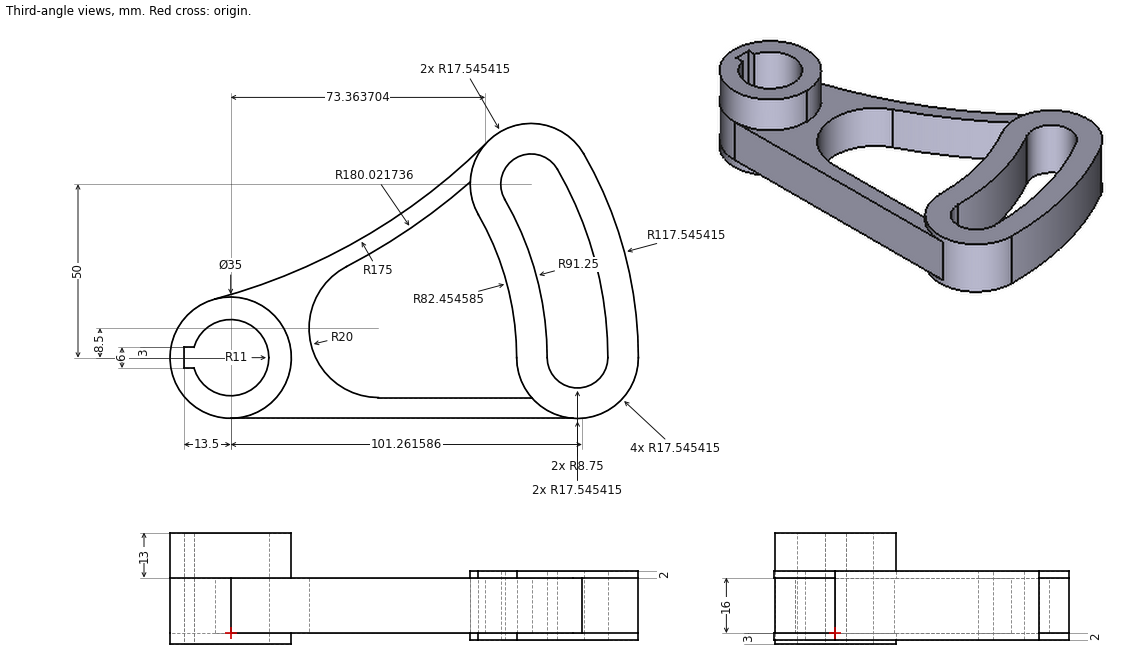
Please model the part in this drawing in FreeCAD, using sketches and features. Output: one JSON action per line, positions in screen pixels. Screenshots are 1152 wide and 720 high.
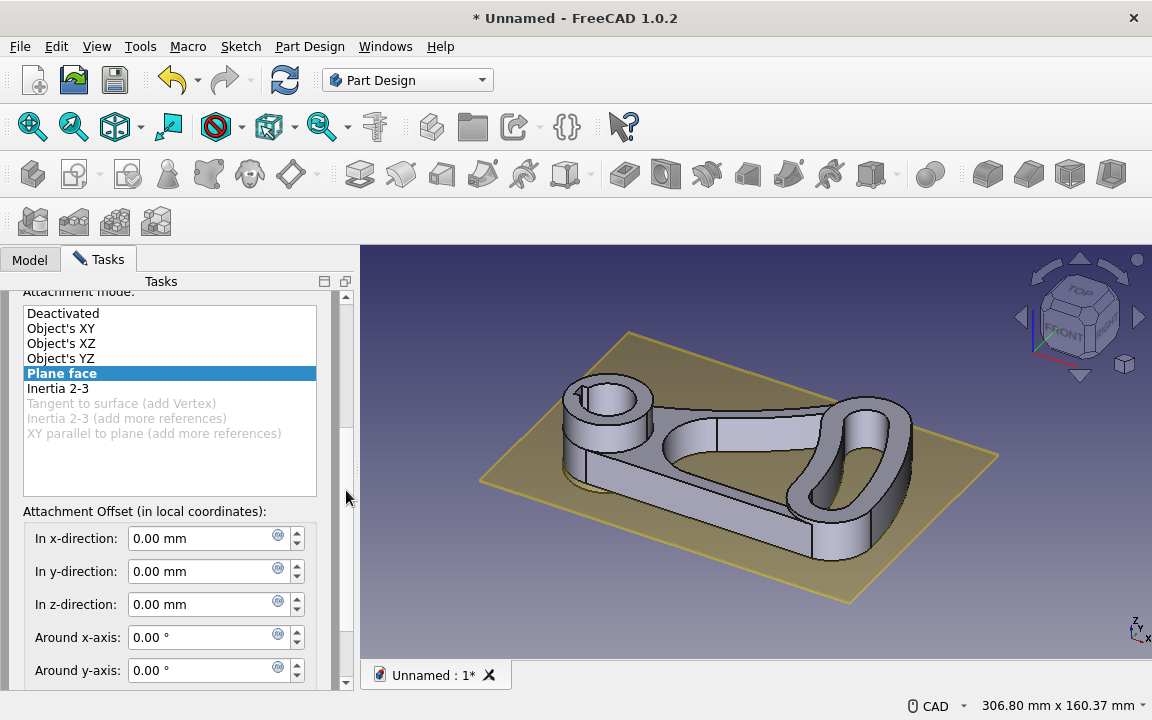
{"action": "triple_click", "coordinate": [210, 604]}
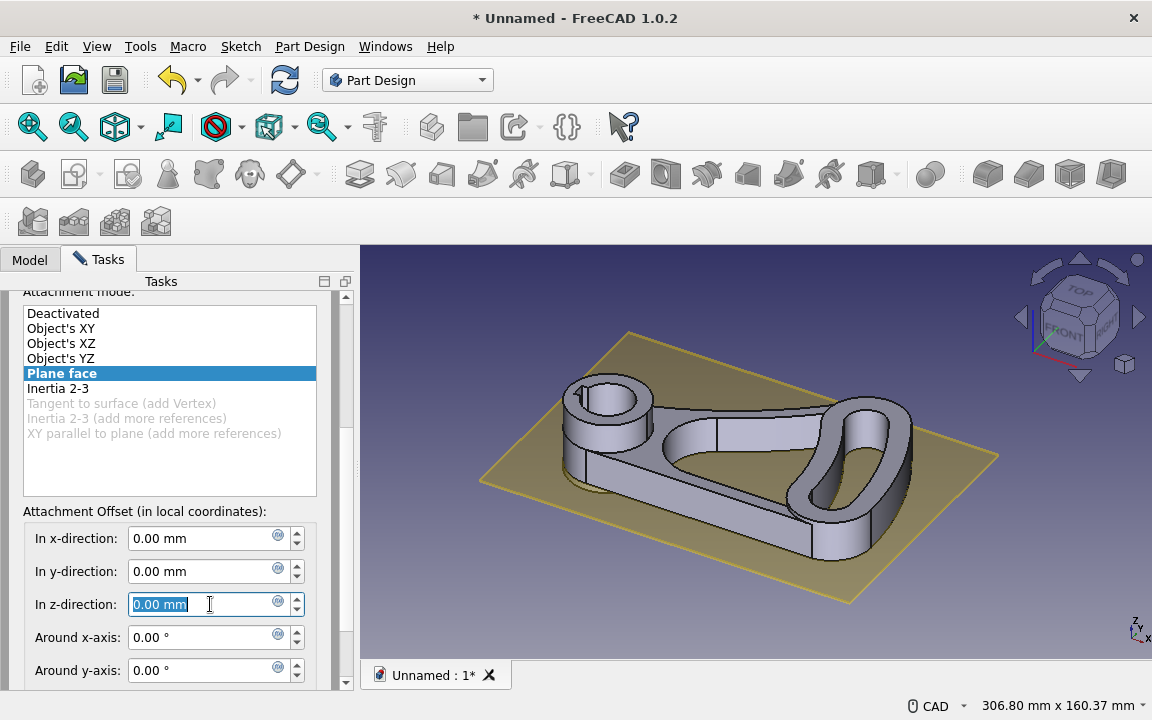
{"action": "type", "text": "-2"}
{"action": "key", "text": "Tab"}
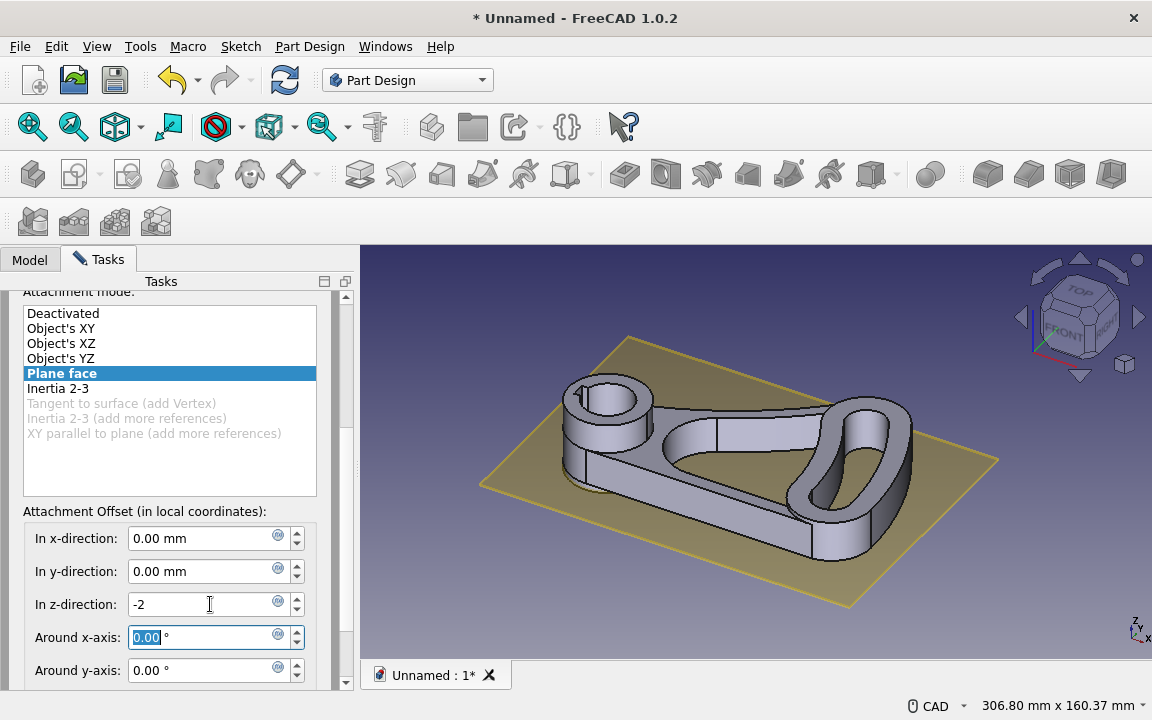
{"action": "scroll", "coordinate": [346, 490], "scroll_direction": "up", "scroll_amount": 5}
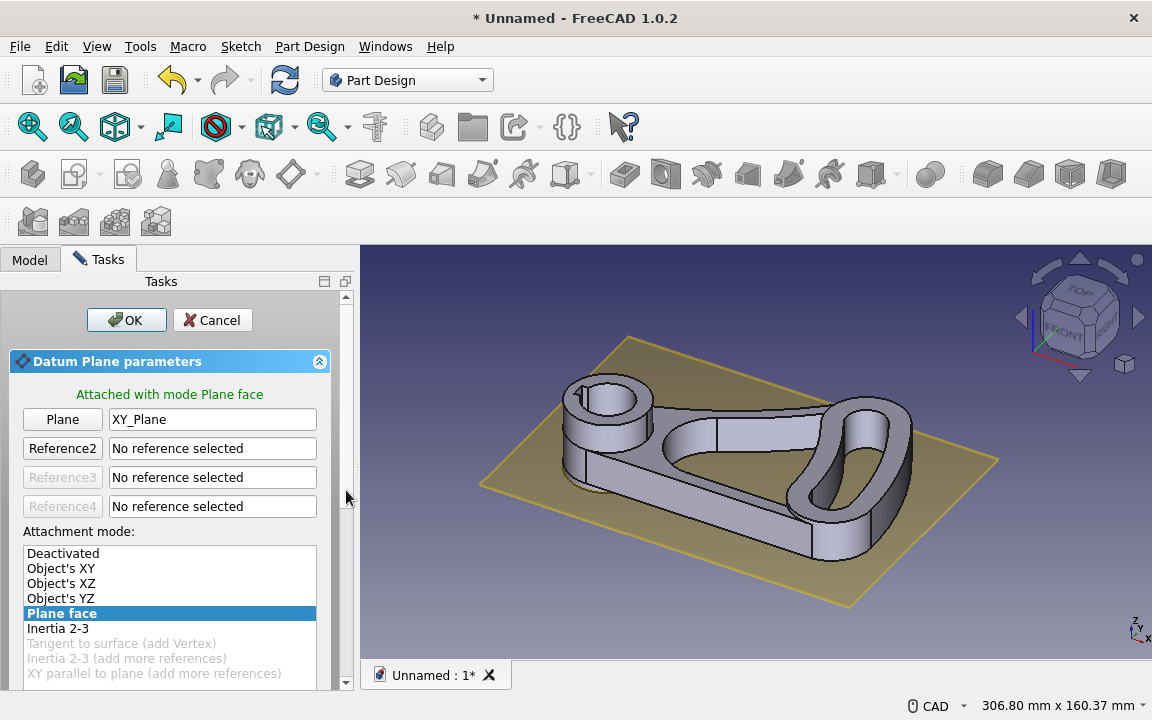
{"action": "left_click", "coordinate": [127, 320]}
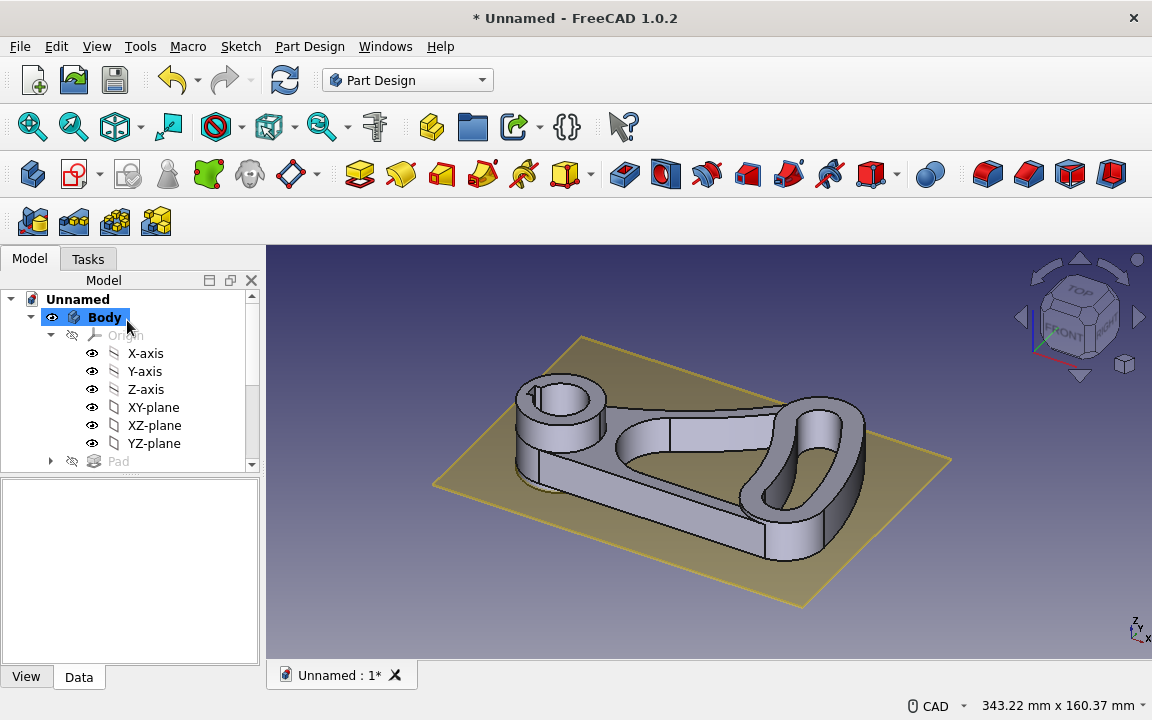
{"action": "scroll", "coordinate": [101, 385], "scroll_direction": "down", "scroll_amount": 3}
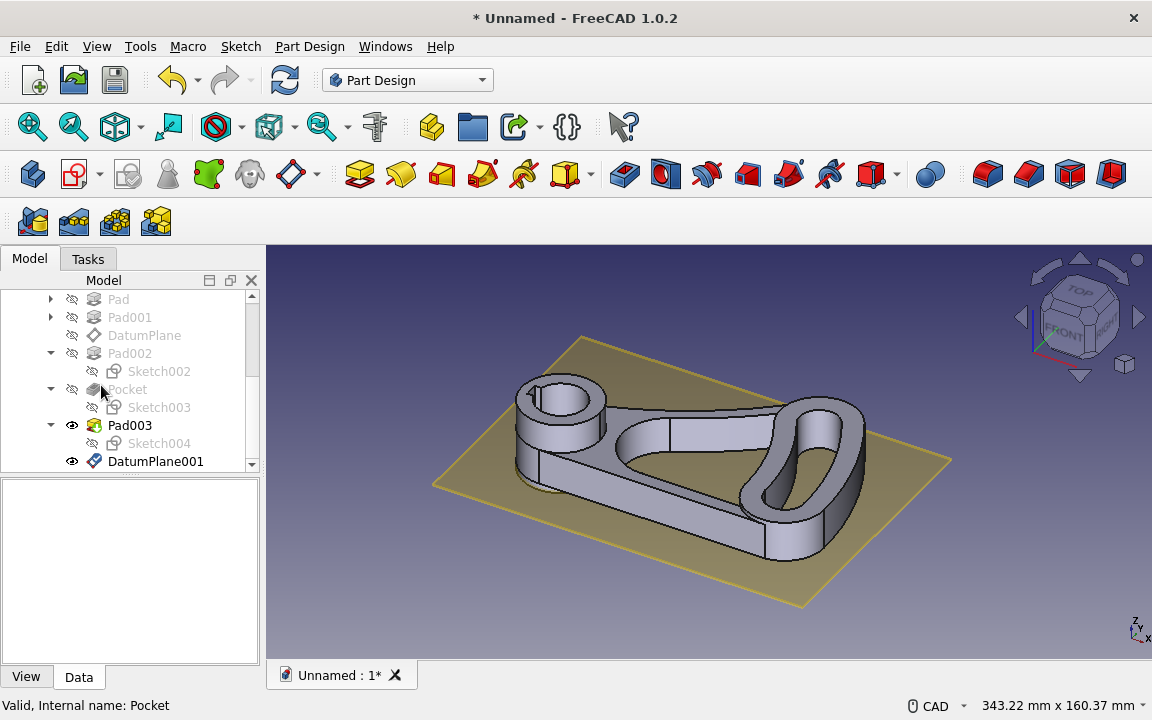
{"action": "left_click", "coordinate": [117, 461]}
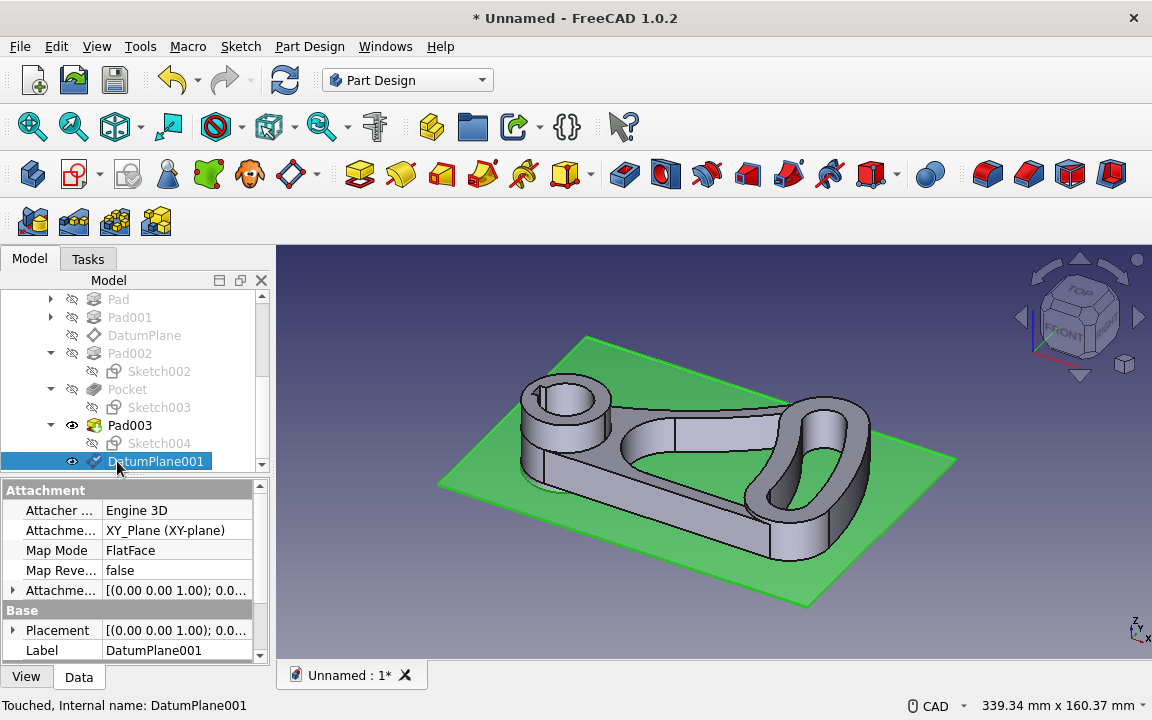
{"action": "left_click", "coordinate": [74, 174]}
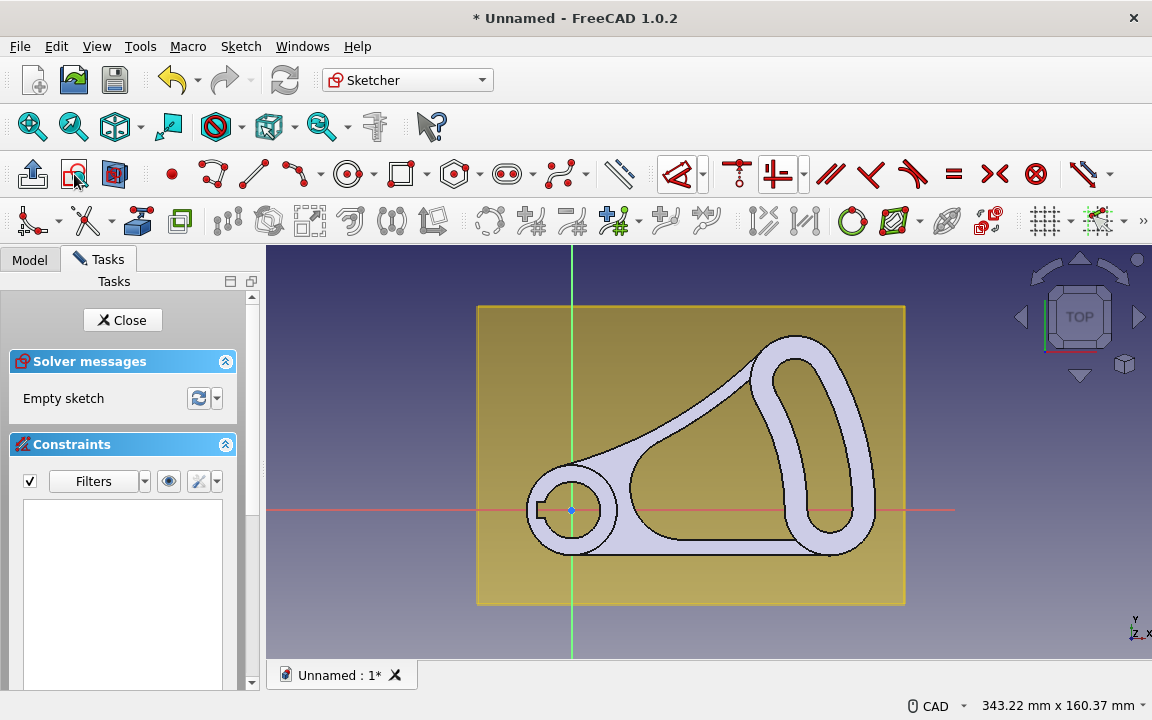
{"action": "left_click", "coordinate": [115, 174]}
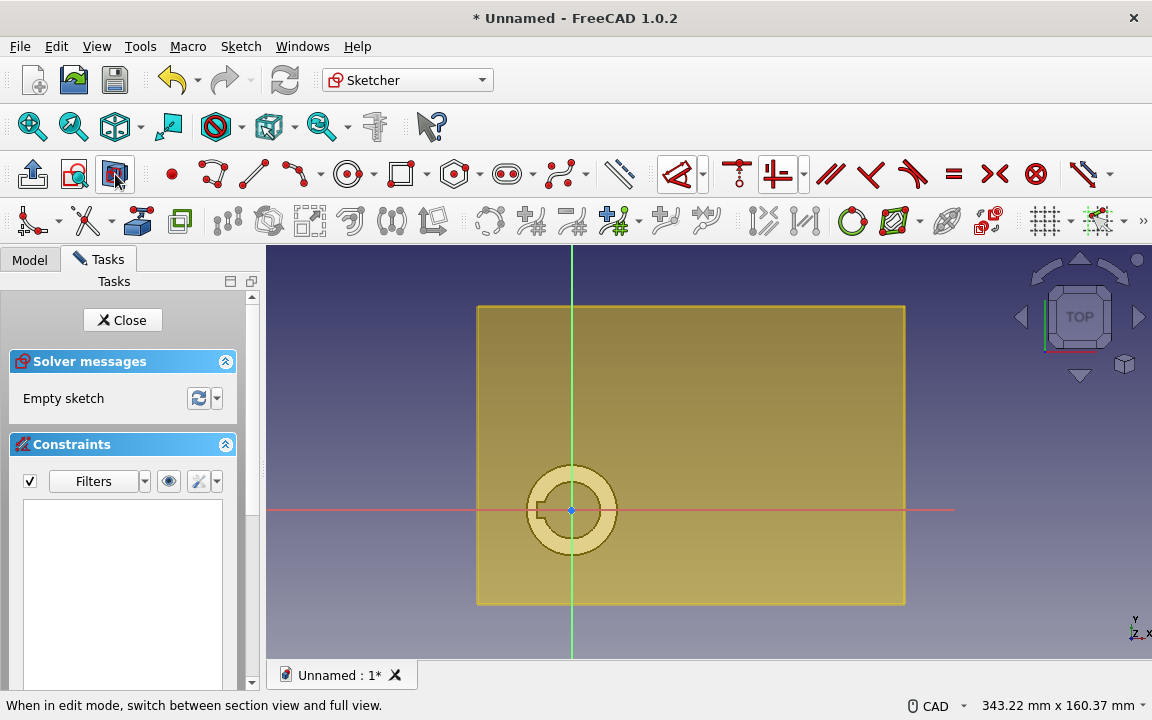
{"action": "left_click", "coordinate": [294, 174]}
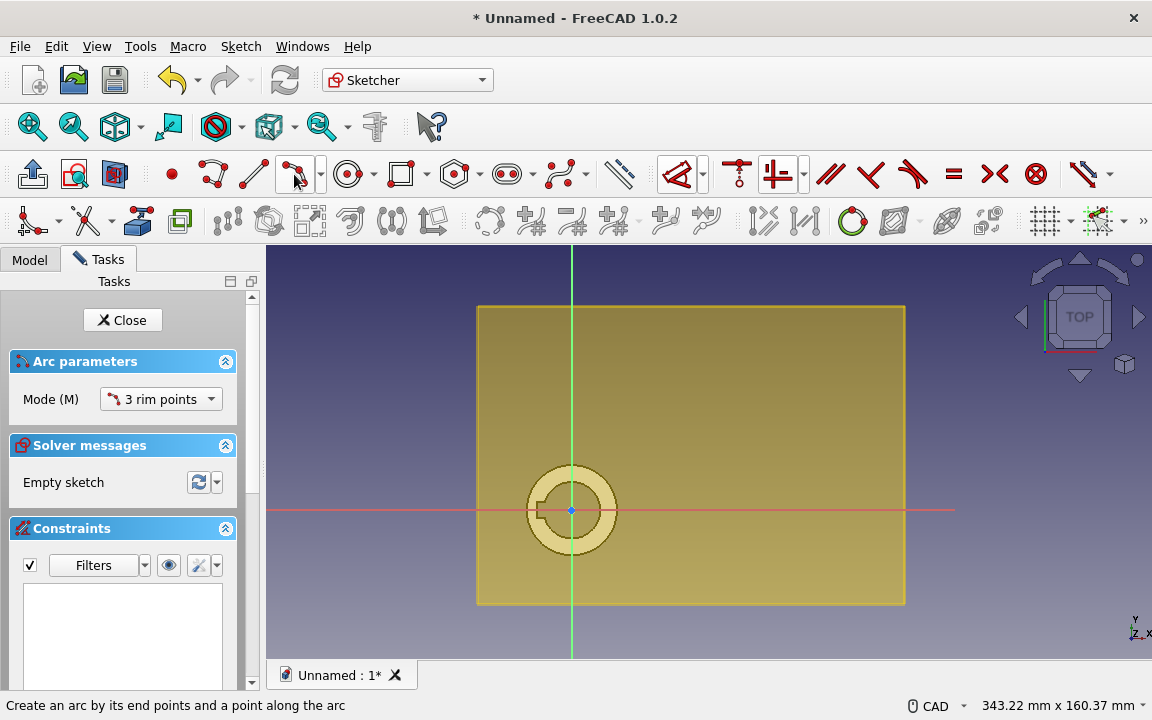
{"action": "left_click", "coordinate": [785, 510]}
{"action": "left_click", "coordinate": [756, 404]}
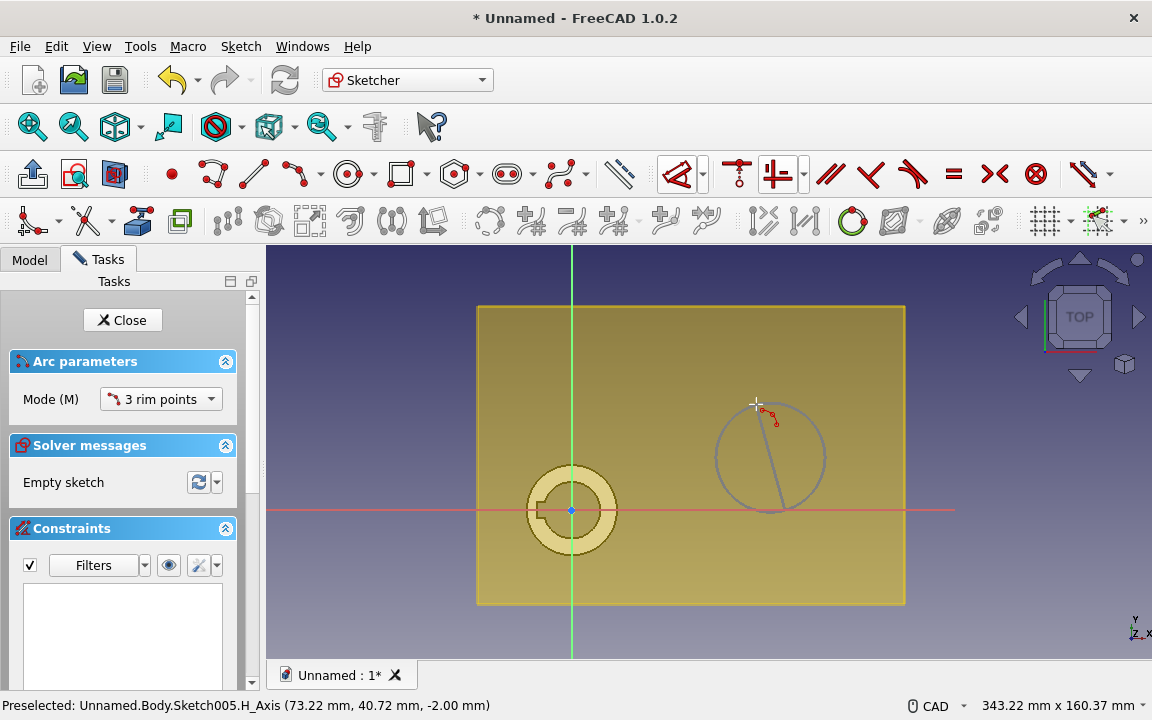
{"action": "scroll", "coordinate": [777, 455], "scroll_direction": "up", "scroll_amount": 4}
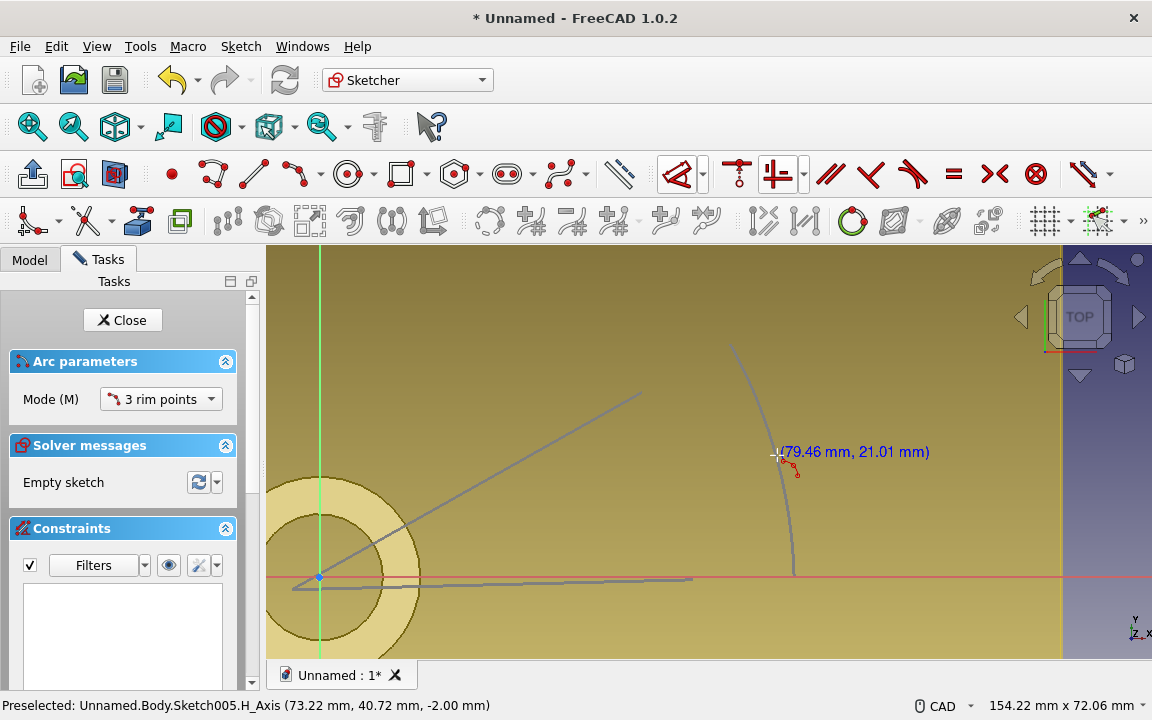
{"action": "left_click", "coordinate": [777, 455]}